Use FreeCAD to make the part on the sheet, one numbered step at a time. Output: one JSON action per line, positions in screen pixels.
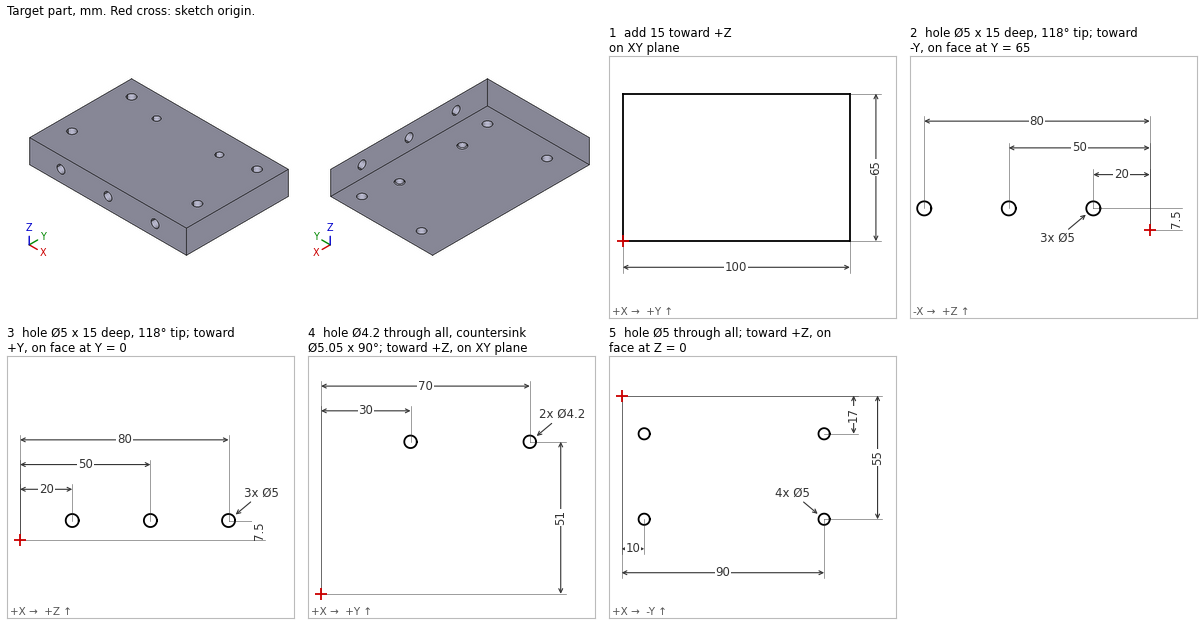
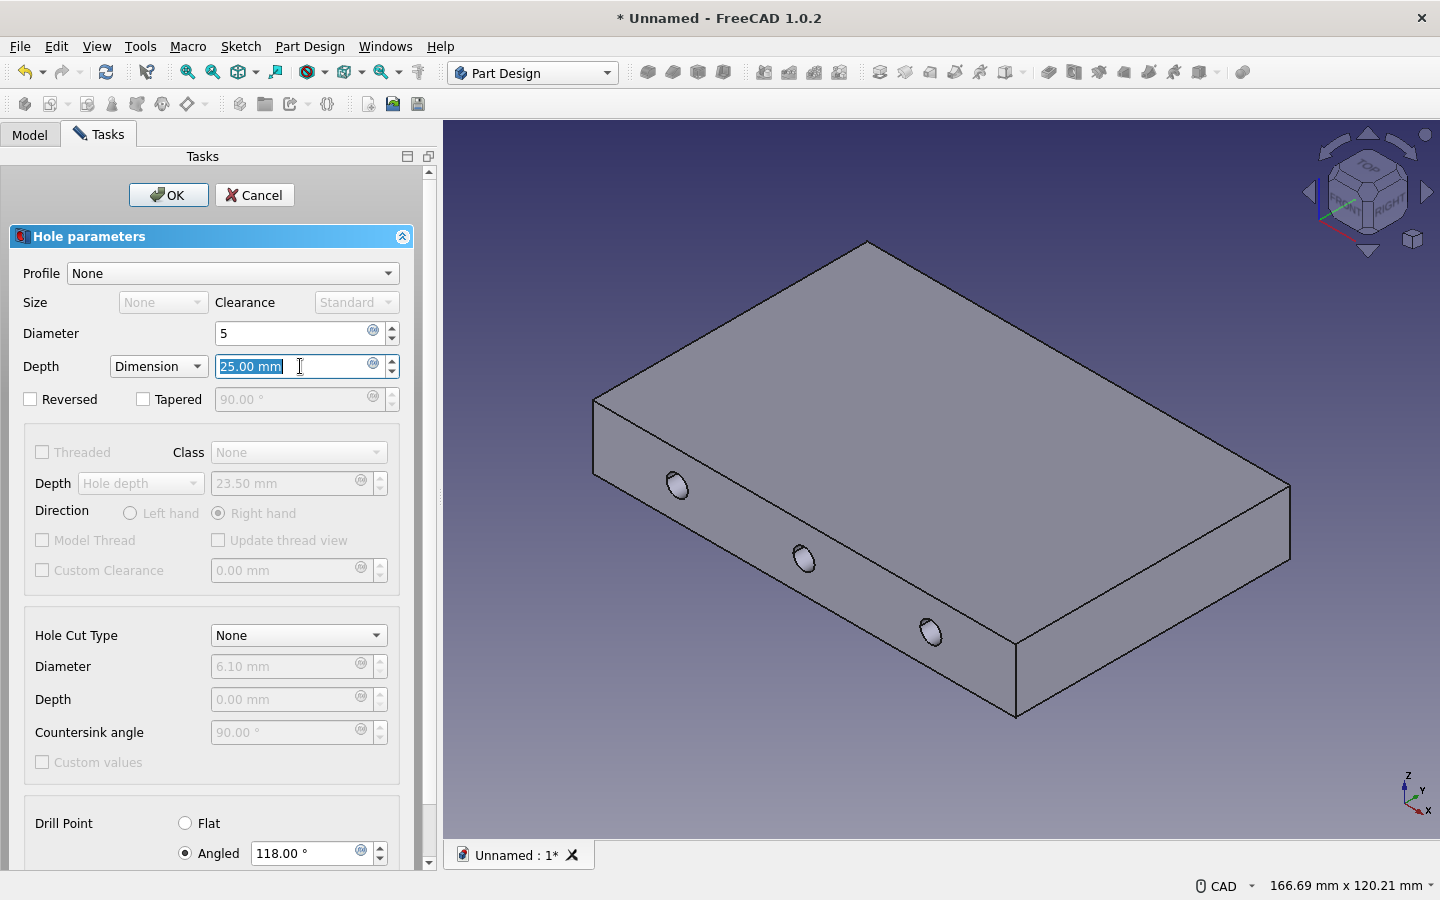
{"action": "type", "text": "15"}
{"action": "key", "text": "Tab"}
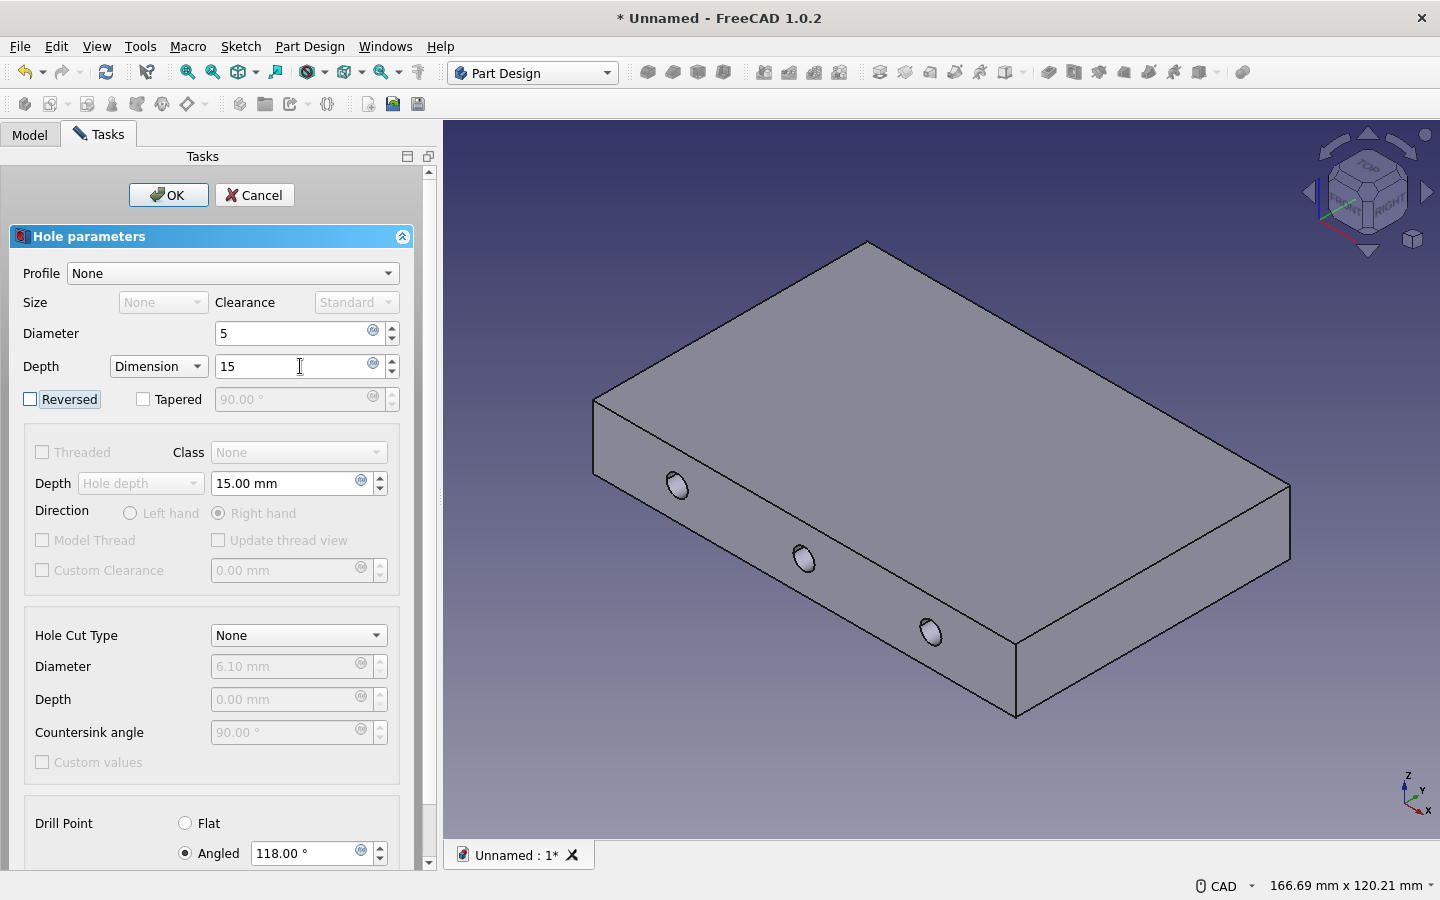
{"action": "left_click", "coordinate": [169, 195]}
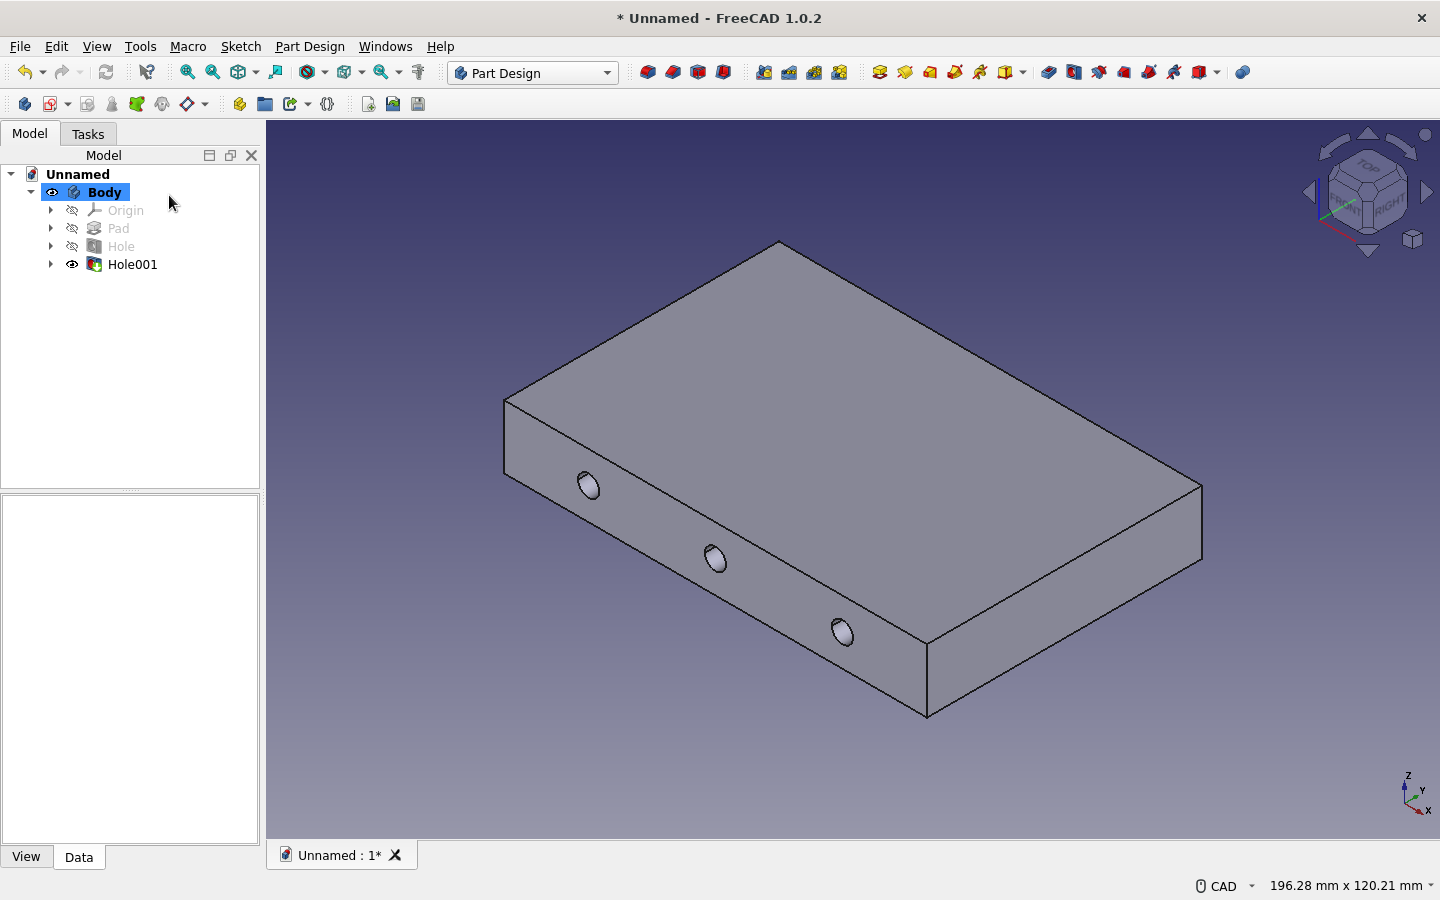
{"action": "left_click", "coordinate": [50, 104]}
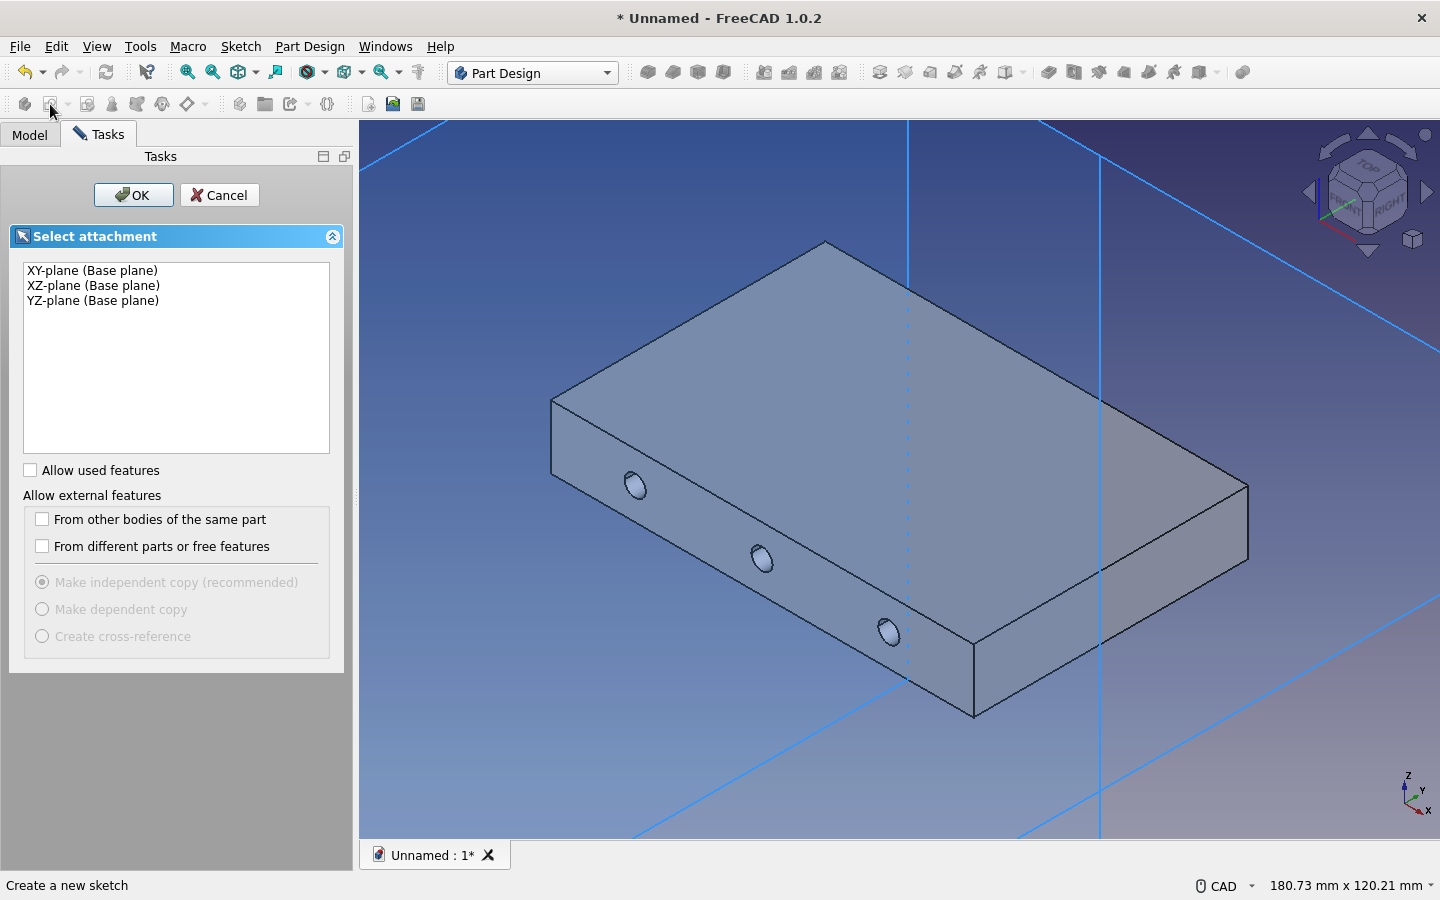
{"action": "left_click", "coordinate": [84, 270]}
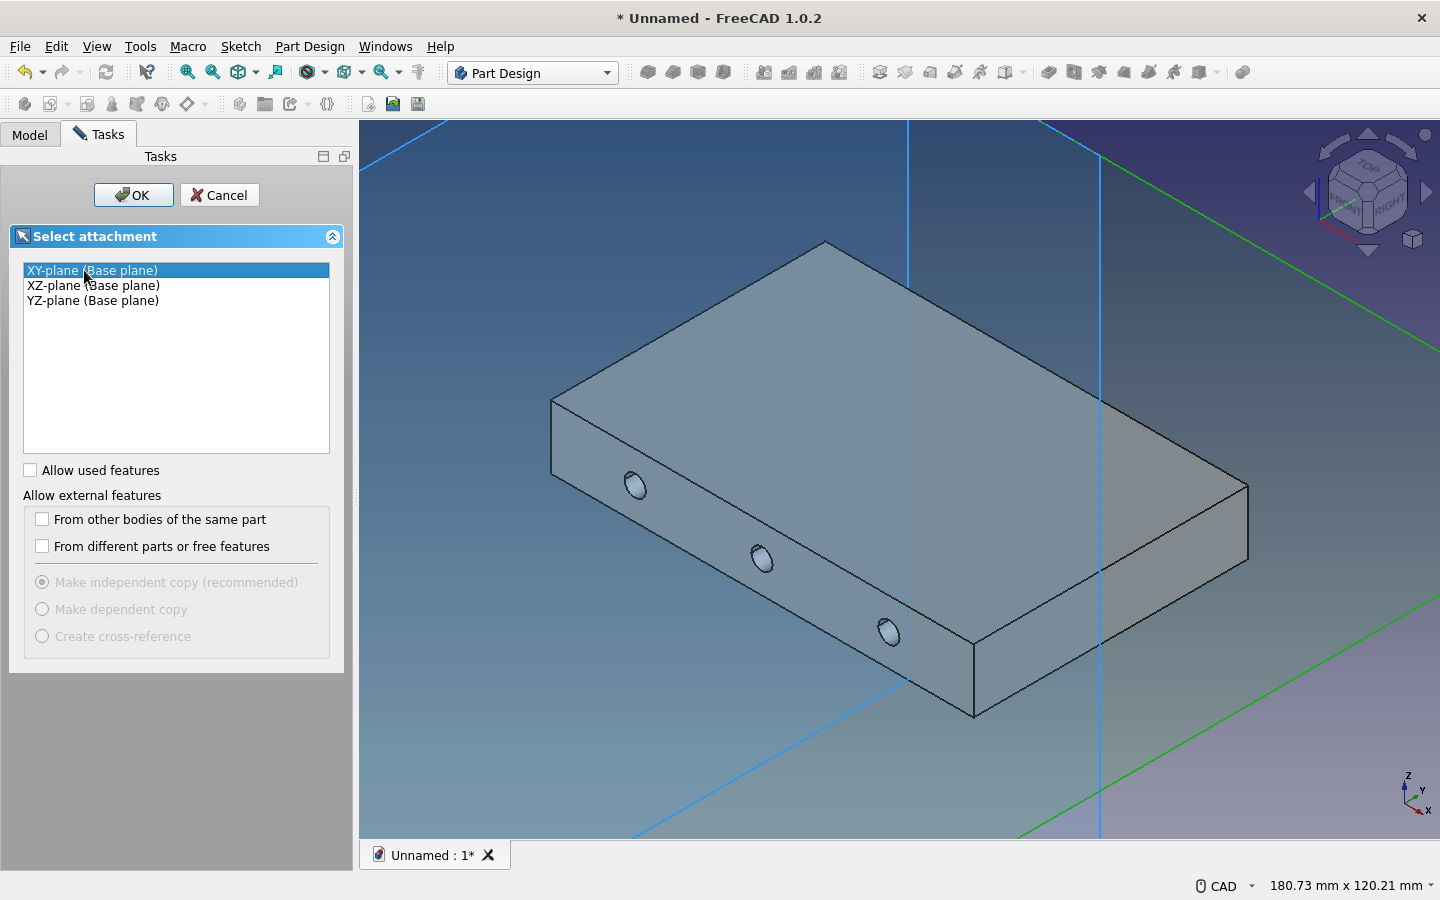
{"action": "left_click", "coordinate": [134, 195]}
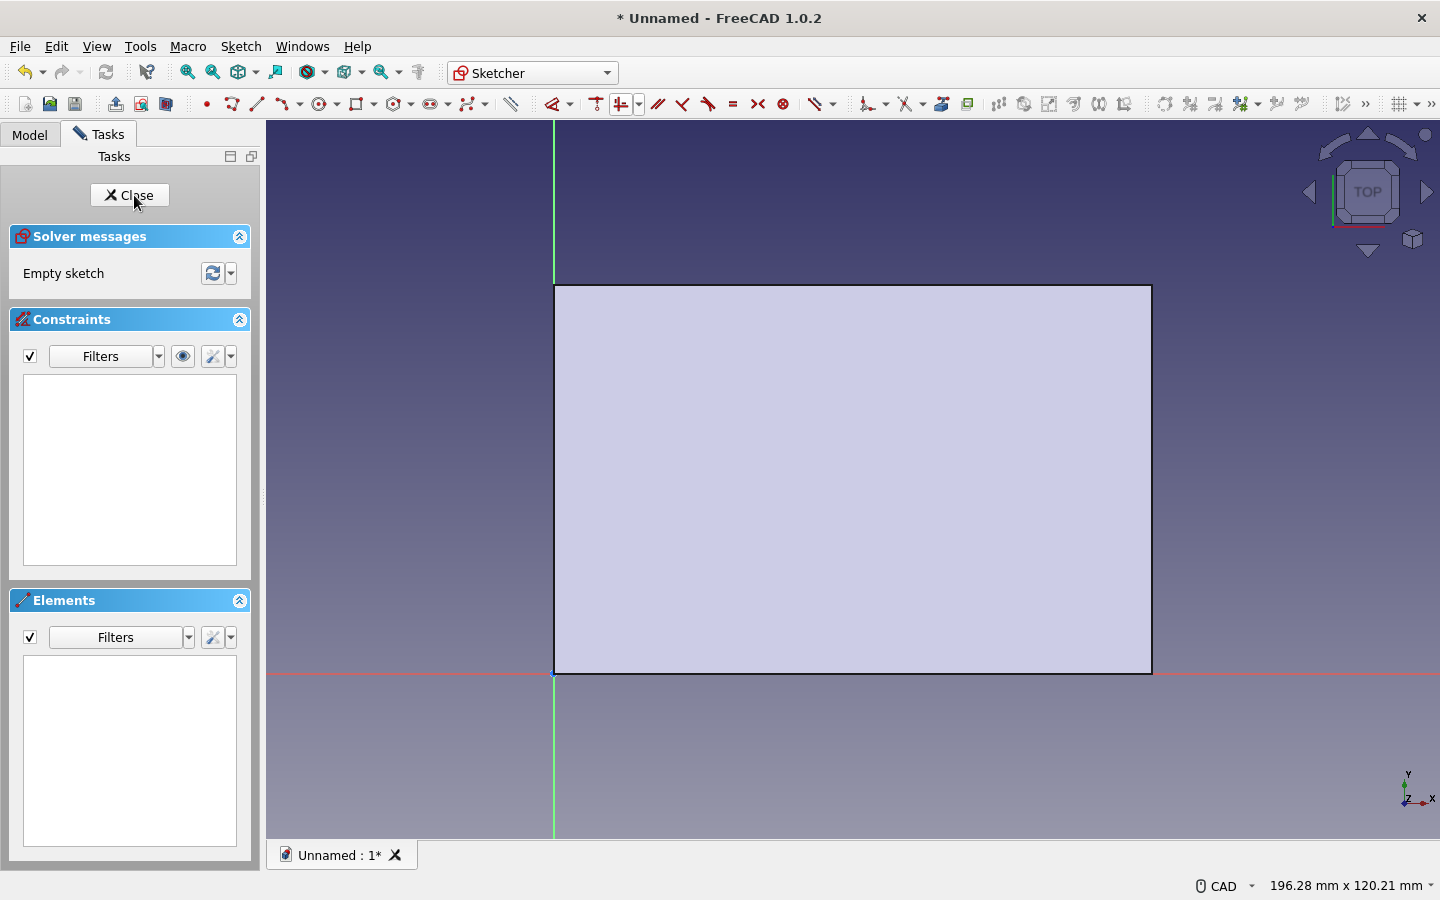
{"action": "left_click", "coordinate": [166, 104]}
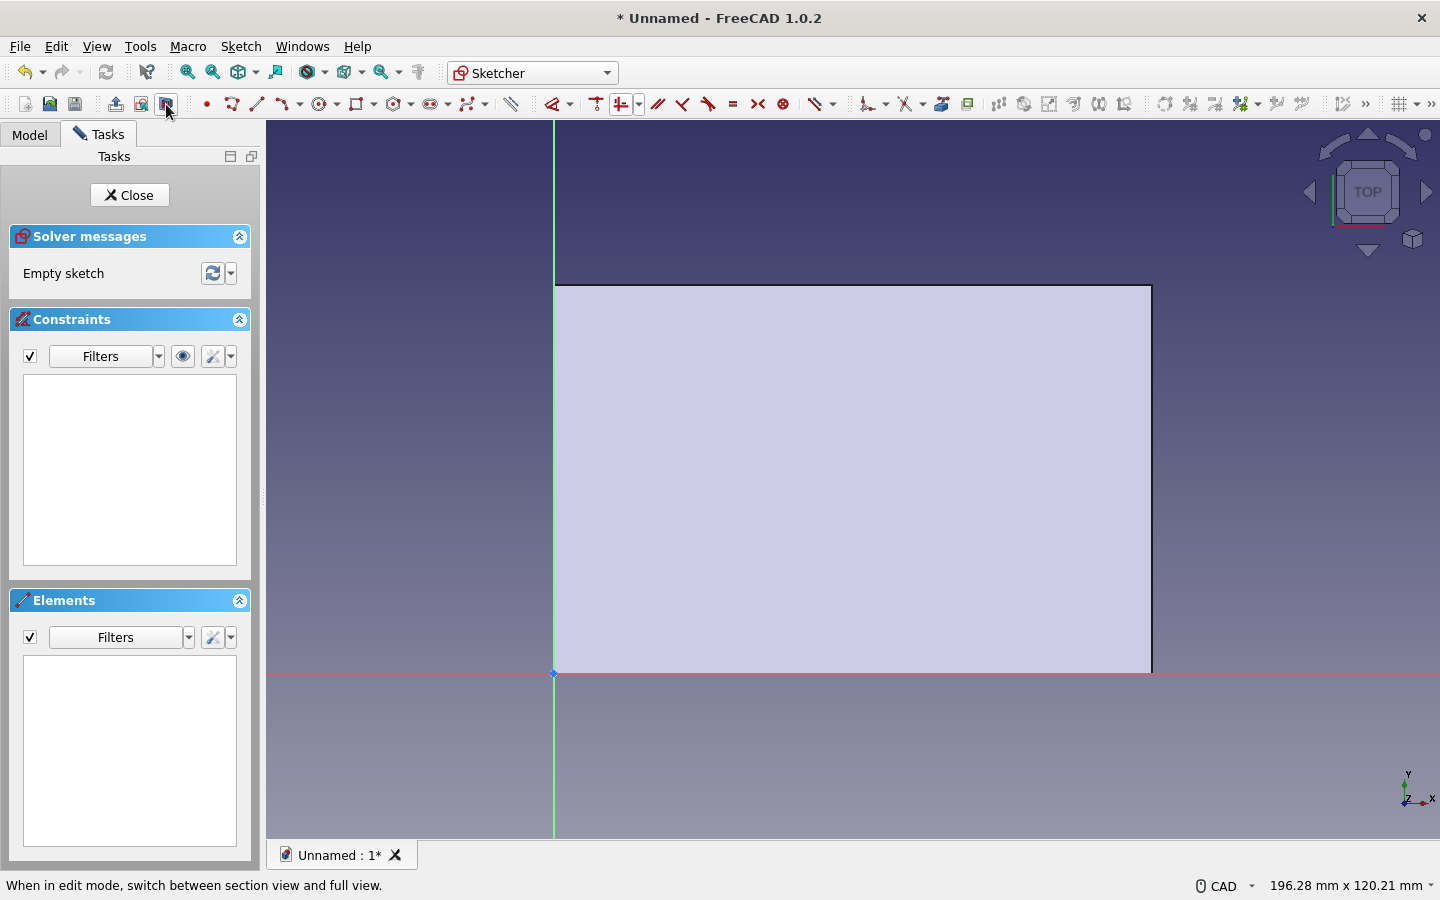
{"action": "scroll", "coordinate": [739, 587], "scroll_direction": "up", "scroll_amount": 2}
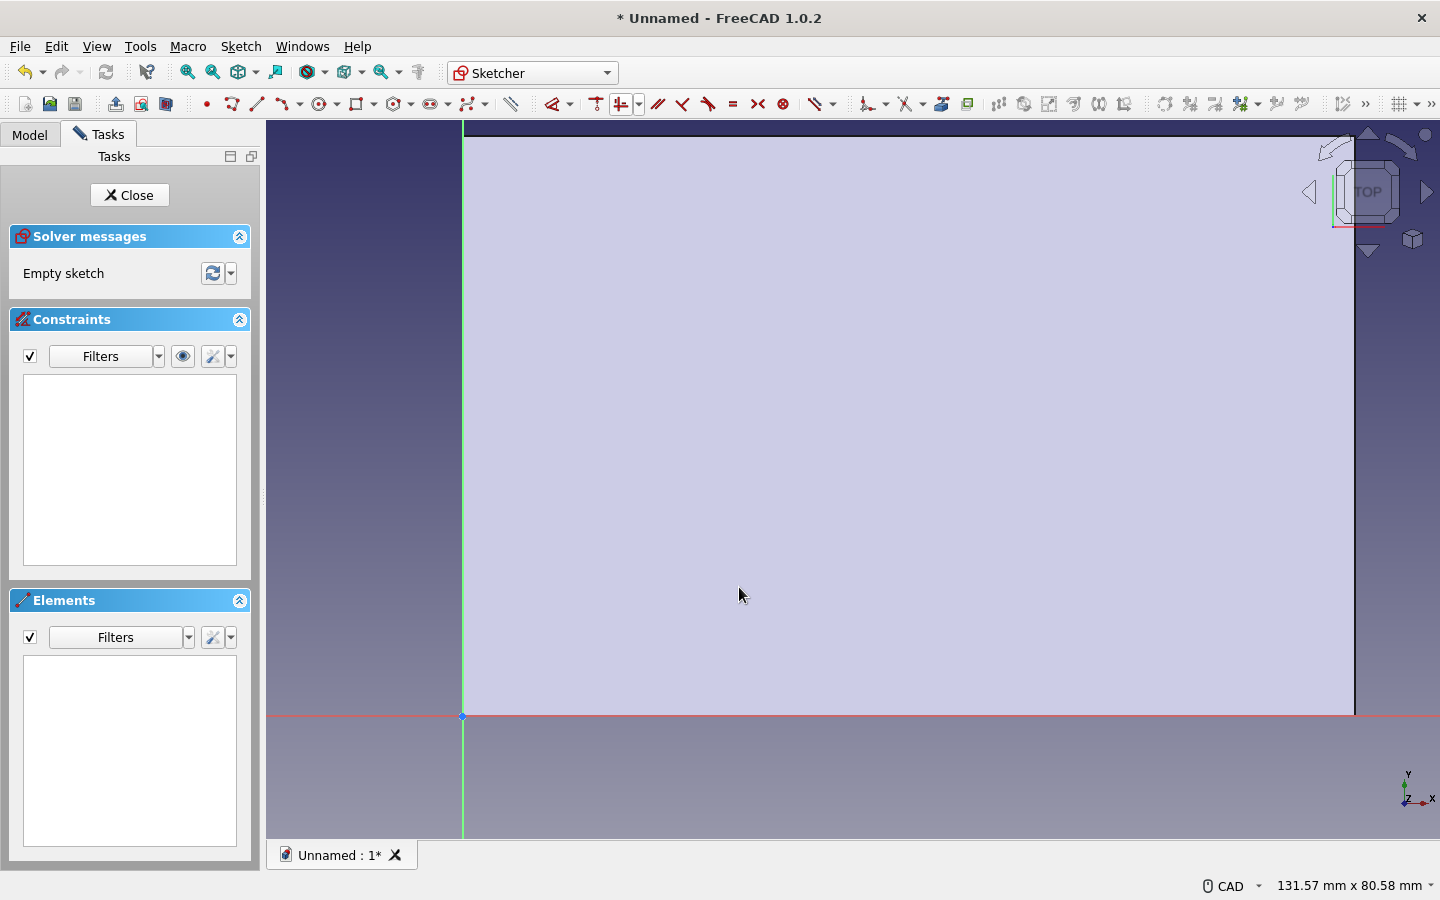
{"action": "left_click", "coordinate": [318, 104]}